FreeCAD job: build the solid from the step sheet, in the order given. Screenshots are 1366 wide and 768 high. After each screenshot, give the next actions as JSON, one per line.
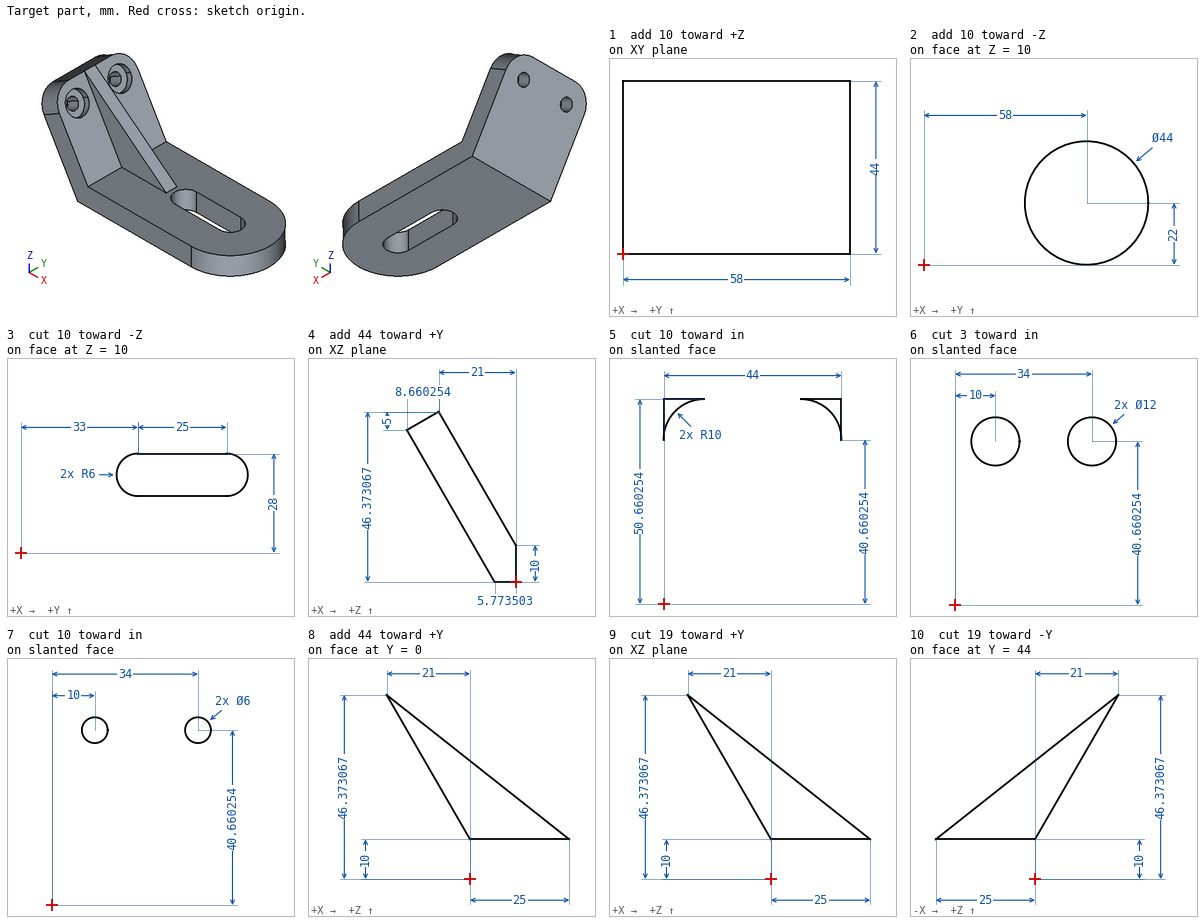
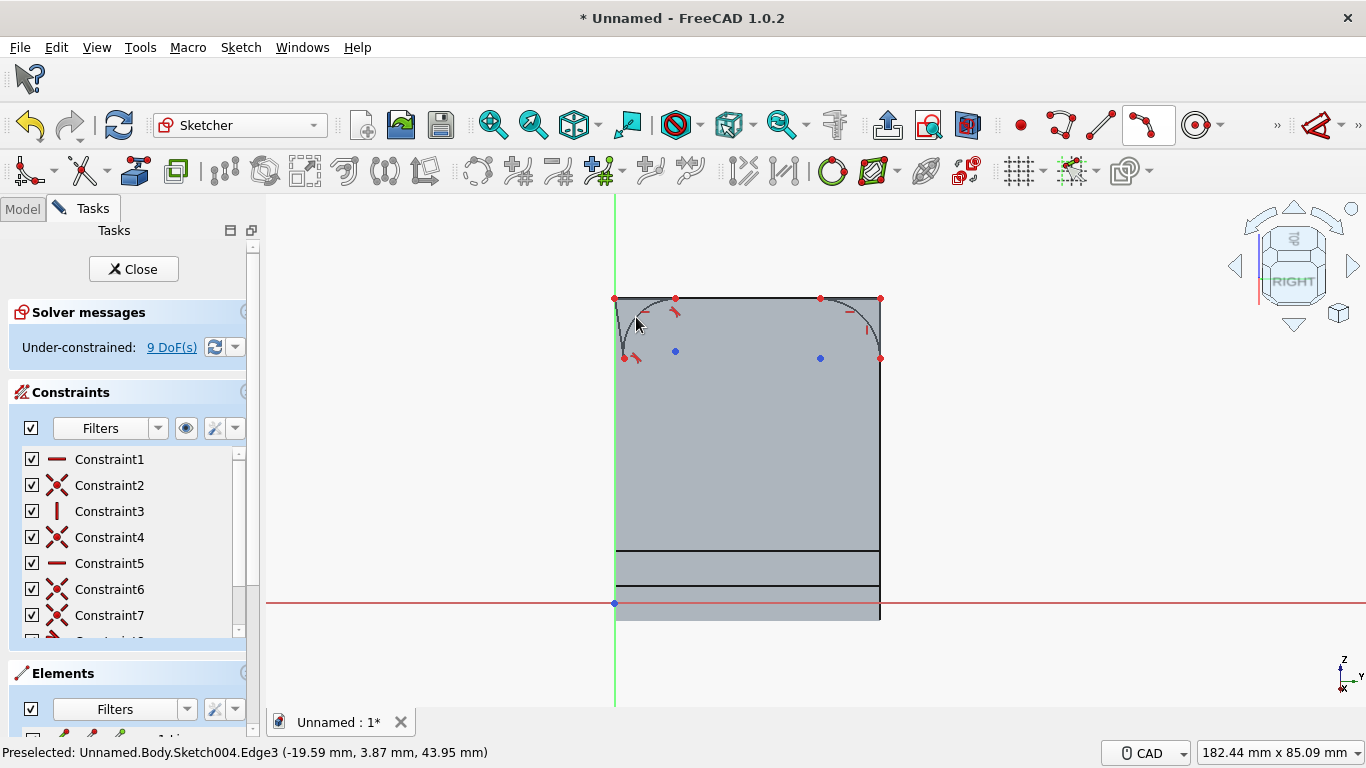
{"action": "left_click", "coordinate": [880, 317]}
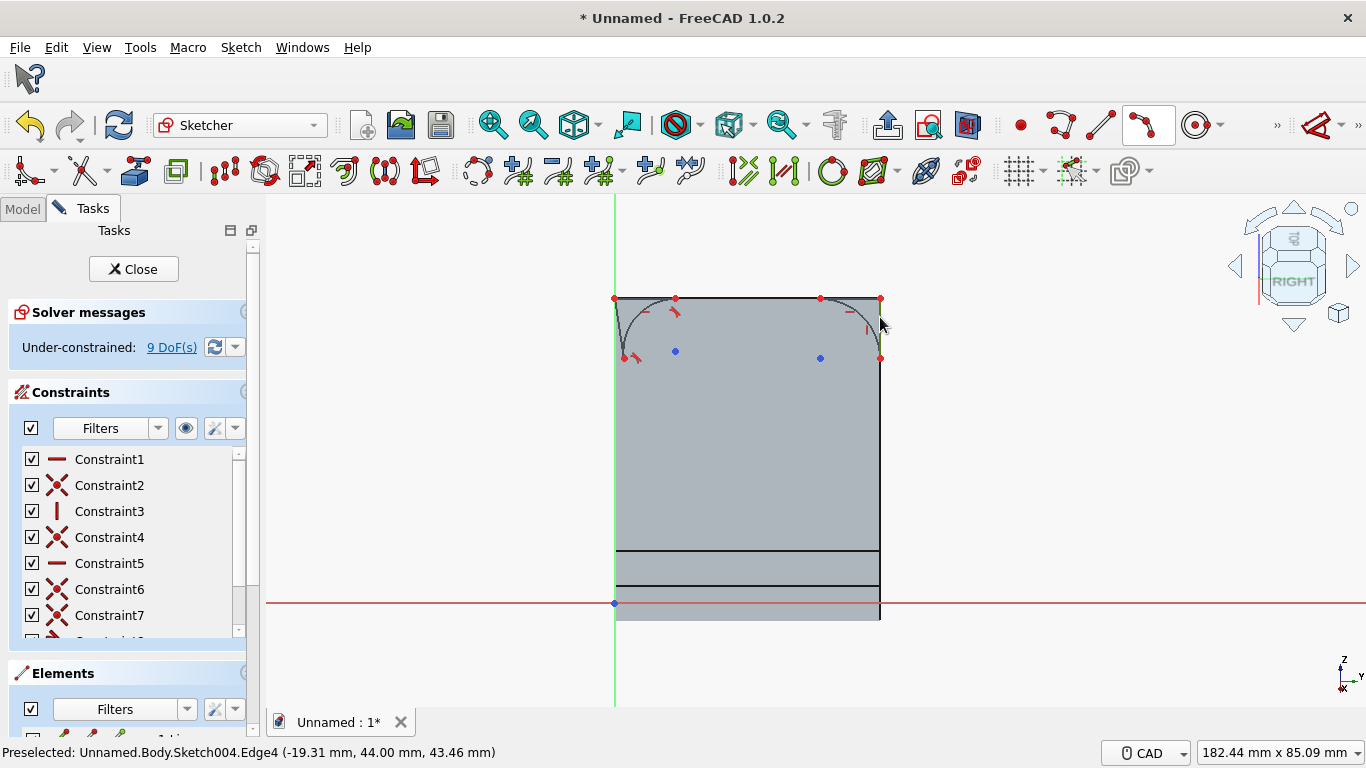
{"action": "left_click", "coordinate": [863, 316]}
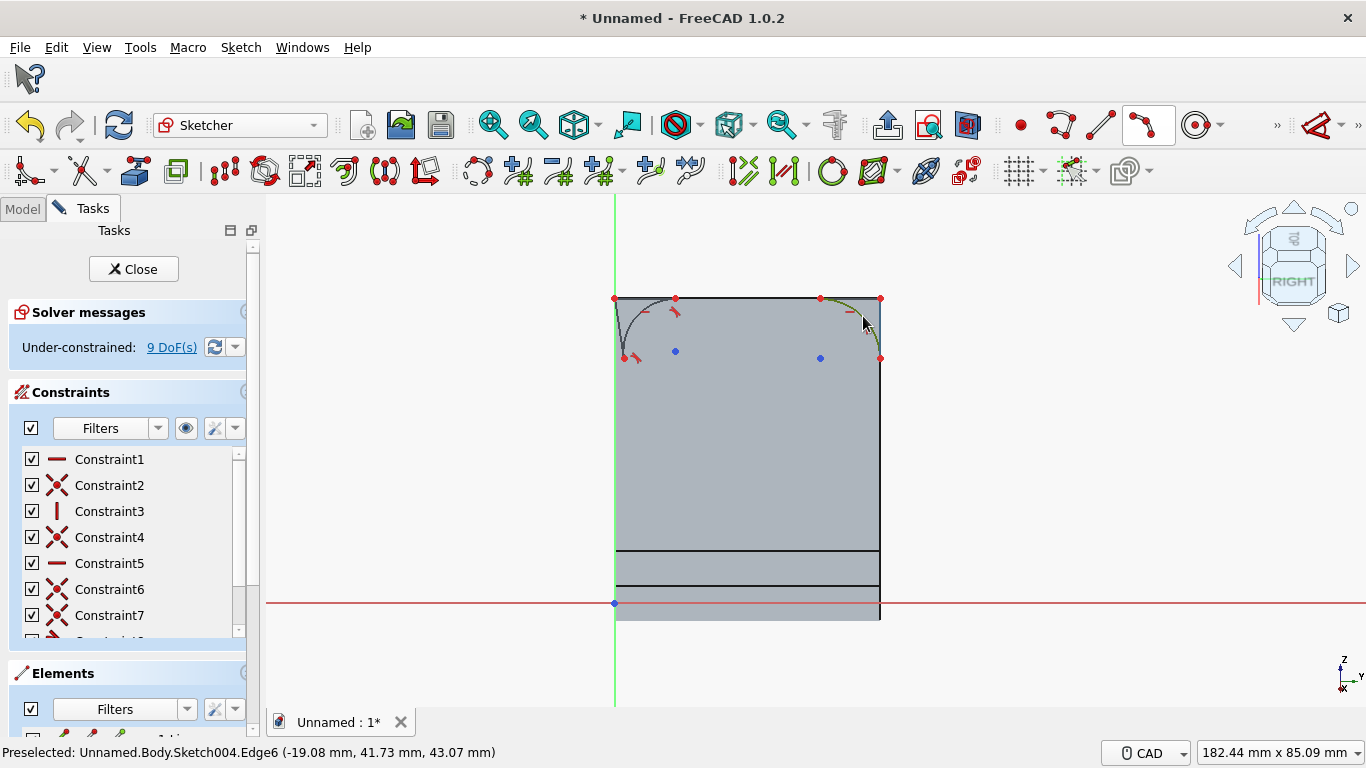
{"action": "key", "text": "t"}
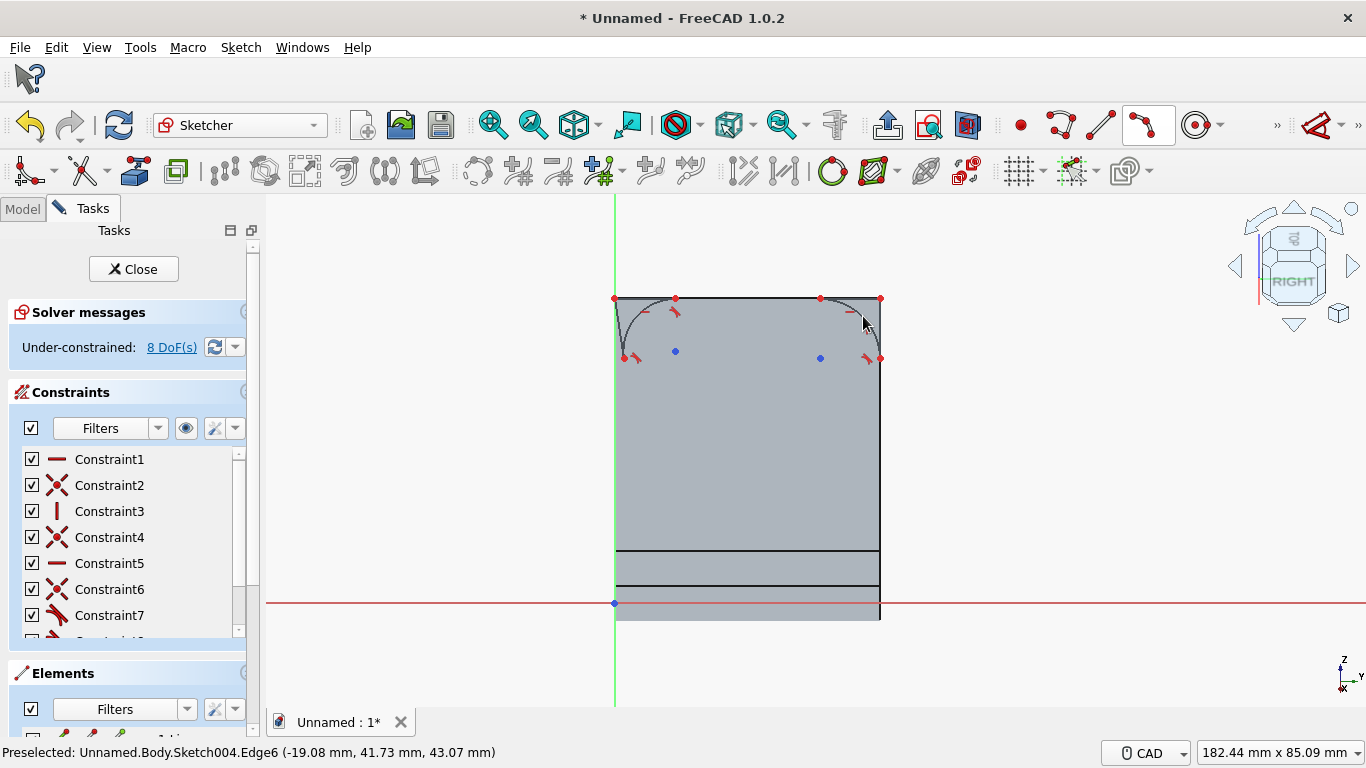
{"action": "left_click", "coordinate": [862, 299]}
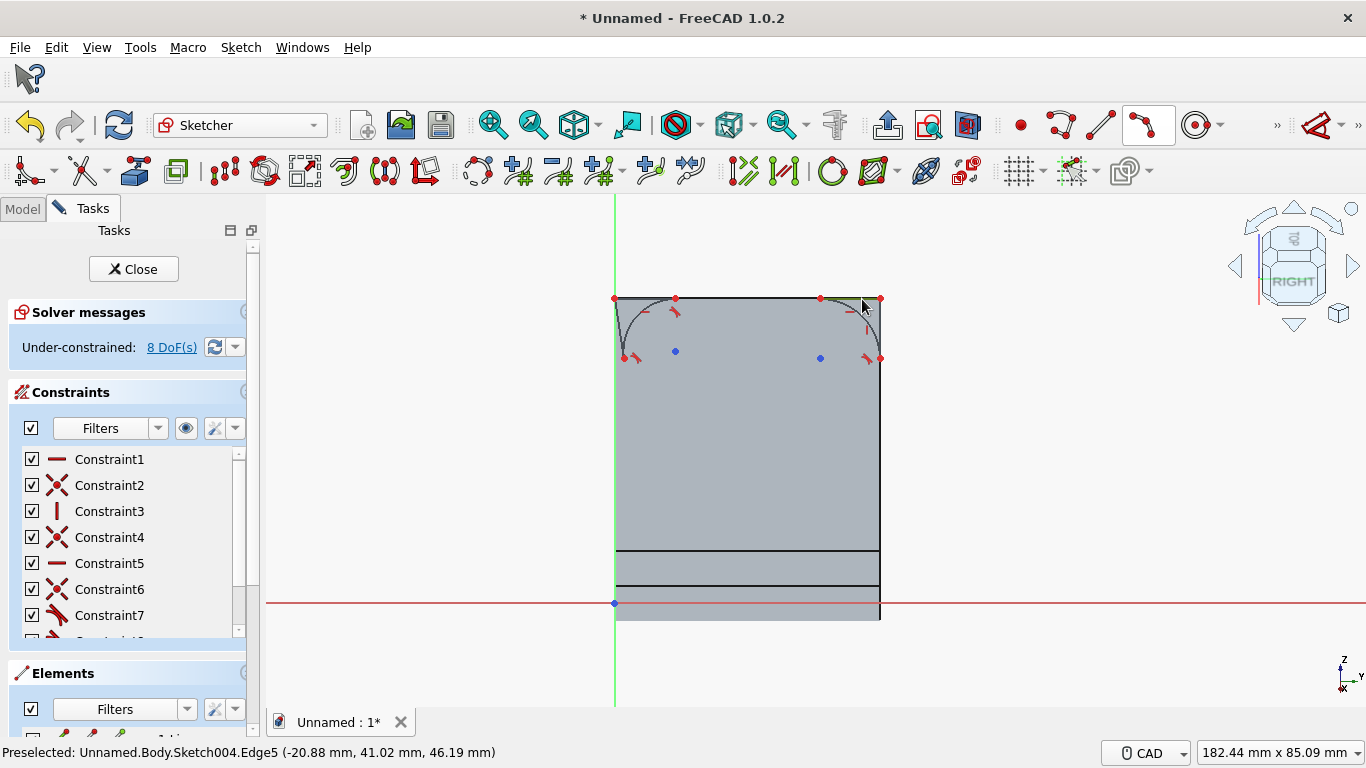
{"action": "left_click", "coordinate": [862, 317]}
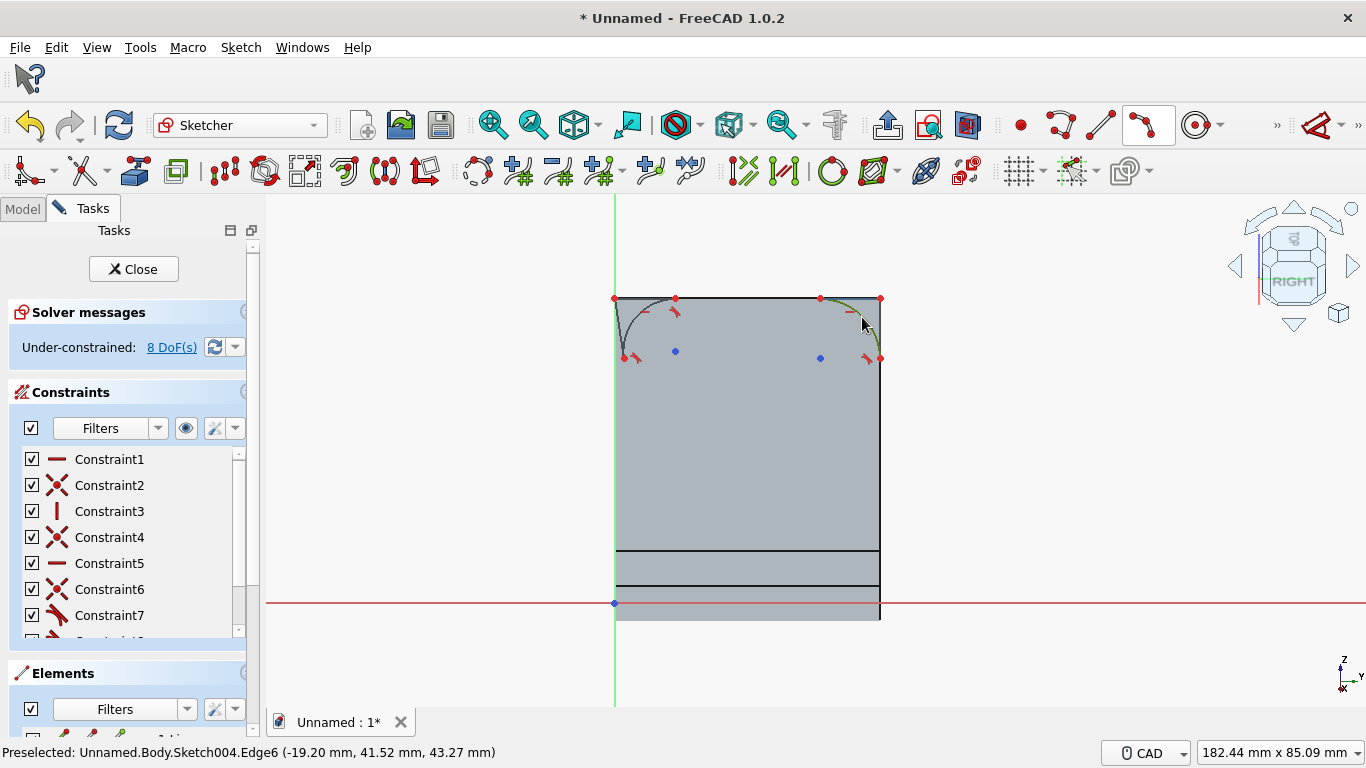
{"action": "key", "text": "t"}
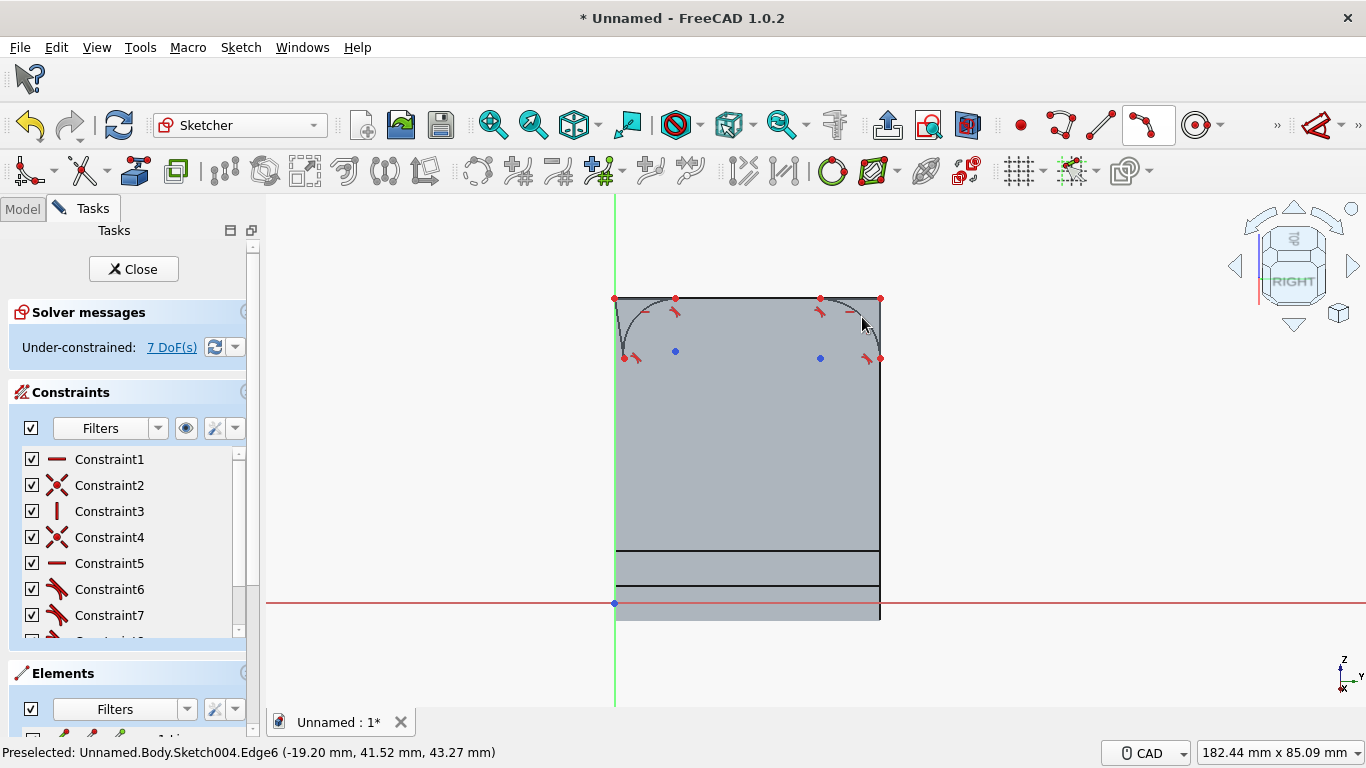
{"action": "left_click", "coordinate": [618, 317]}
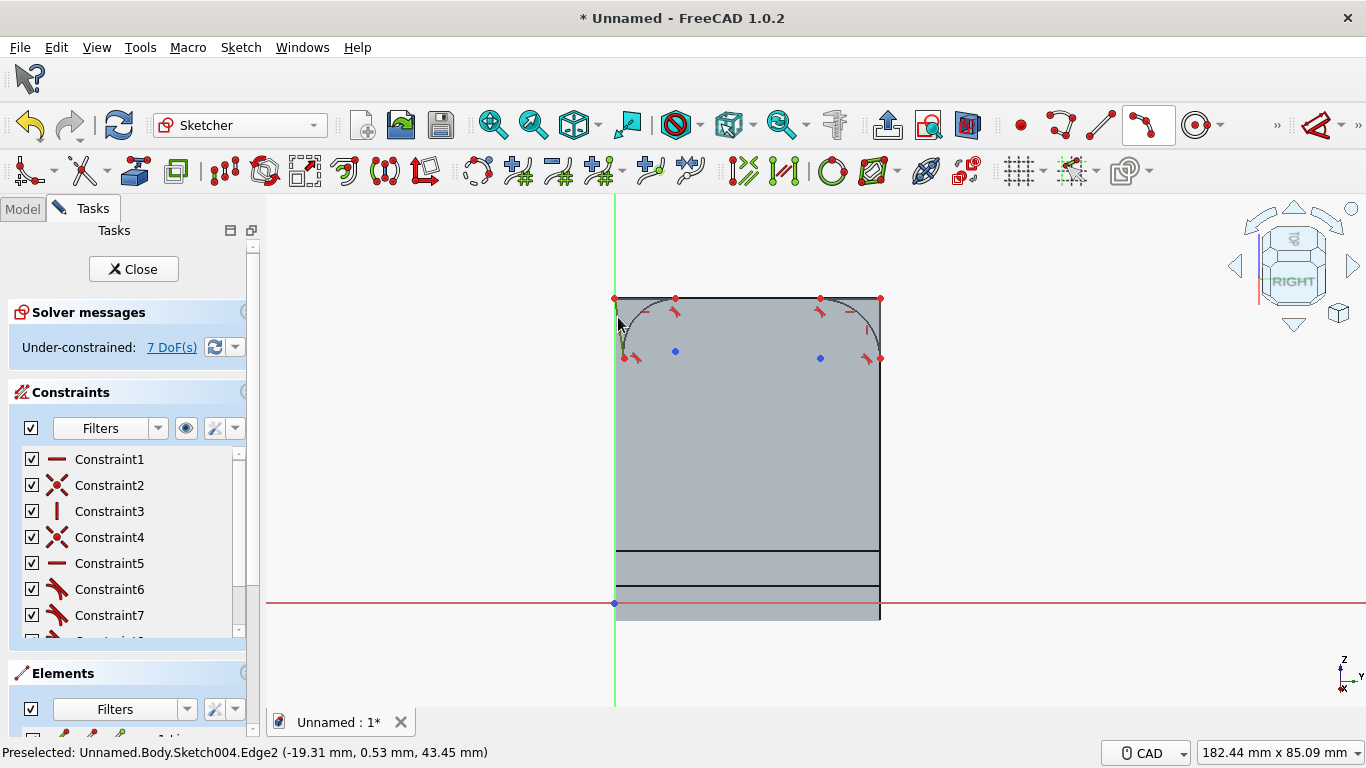
{"action": "key", "text": "v"}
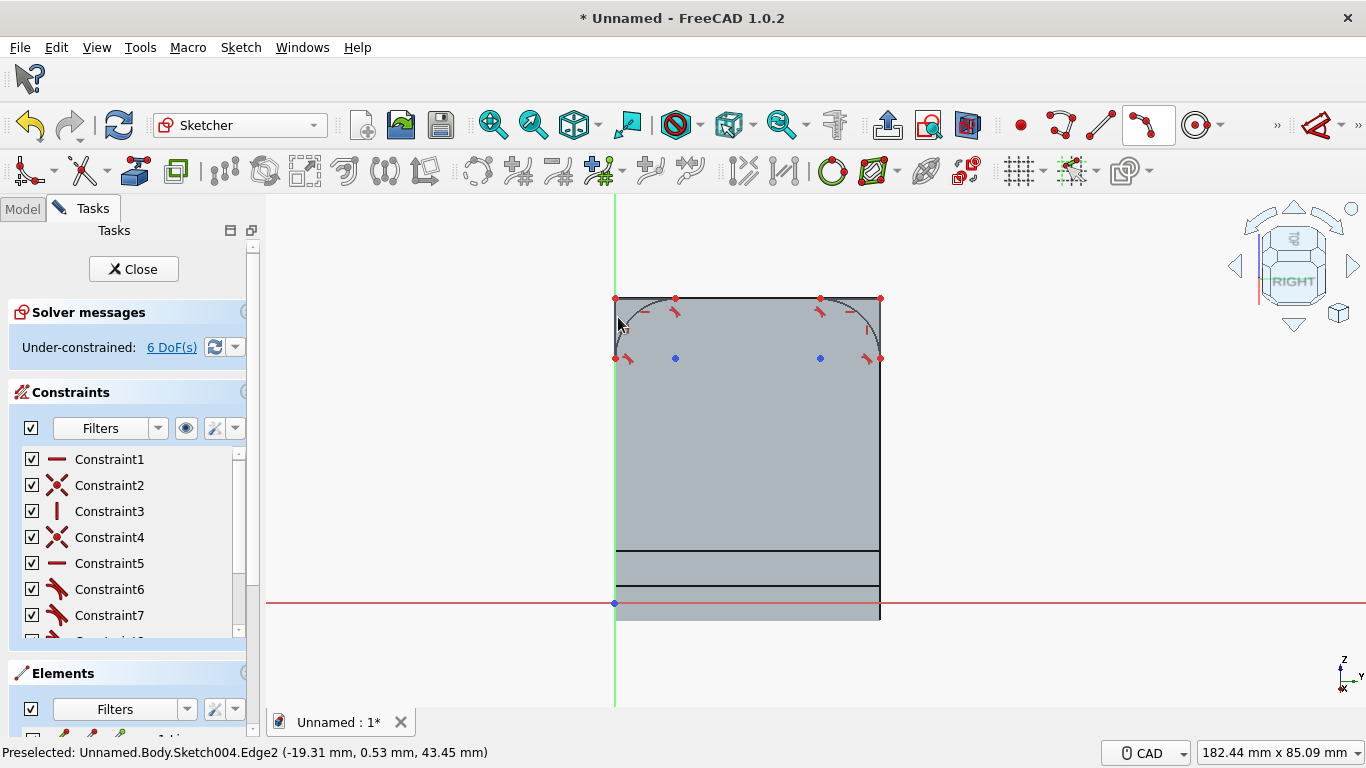
{"action": "left_click", "coordinate": [633, 317]}